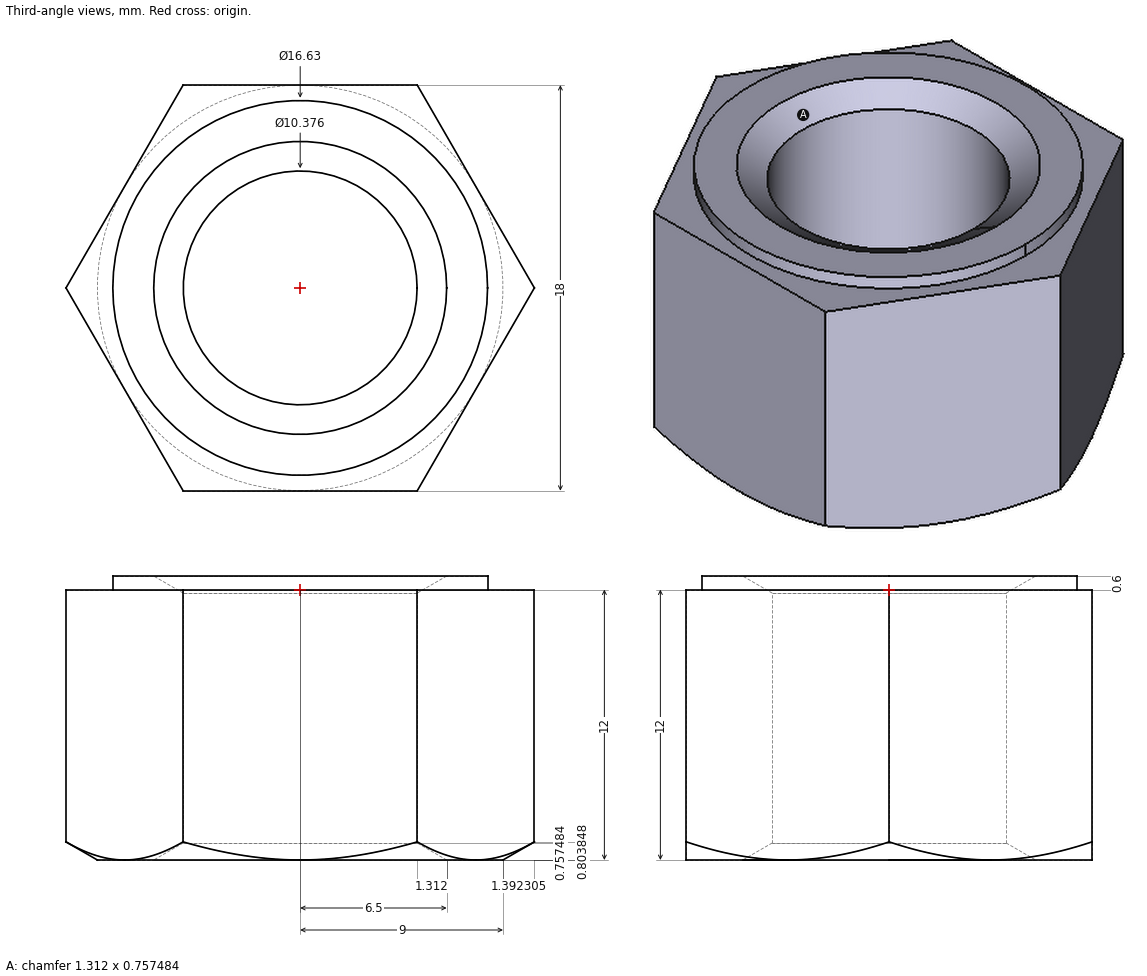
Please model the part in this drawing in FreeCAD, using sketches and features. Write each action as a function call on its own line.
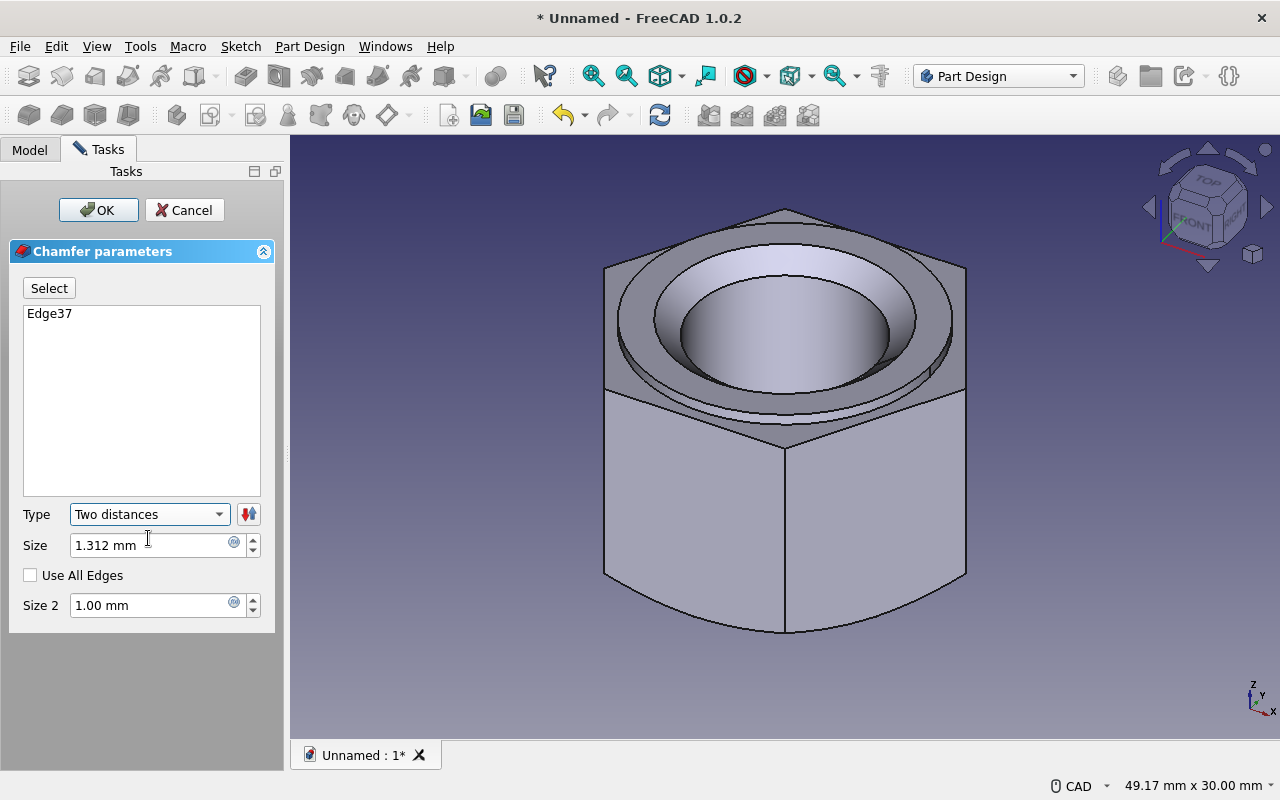
triple_click(158, 606)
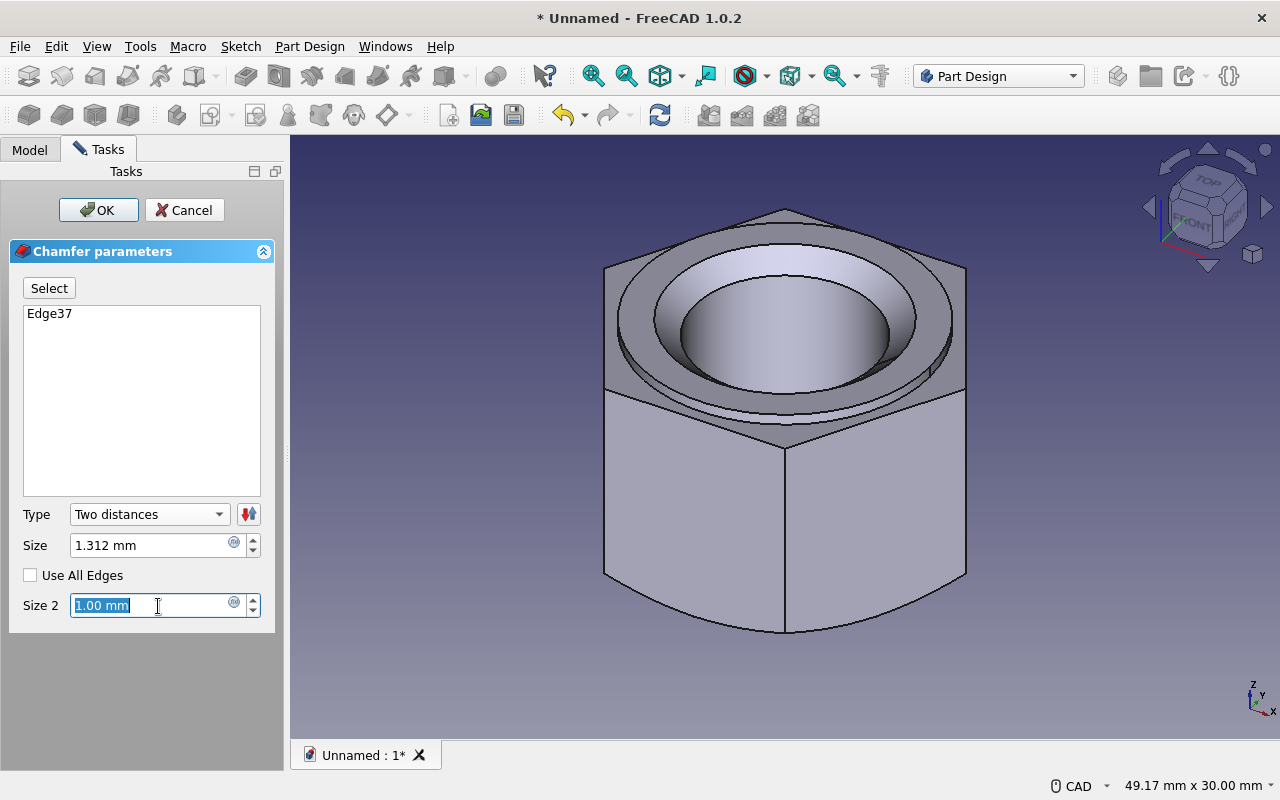
text(0.757484)
key(Tab)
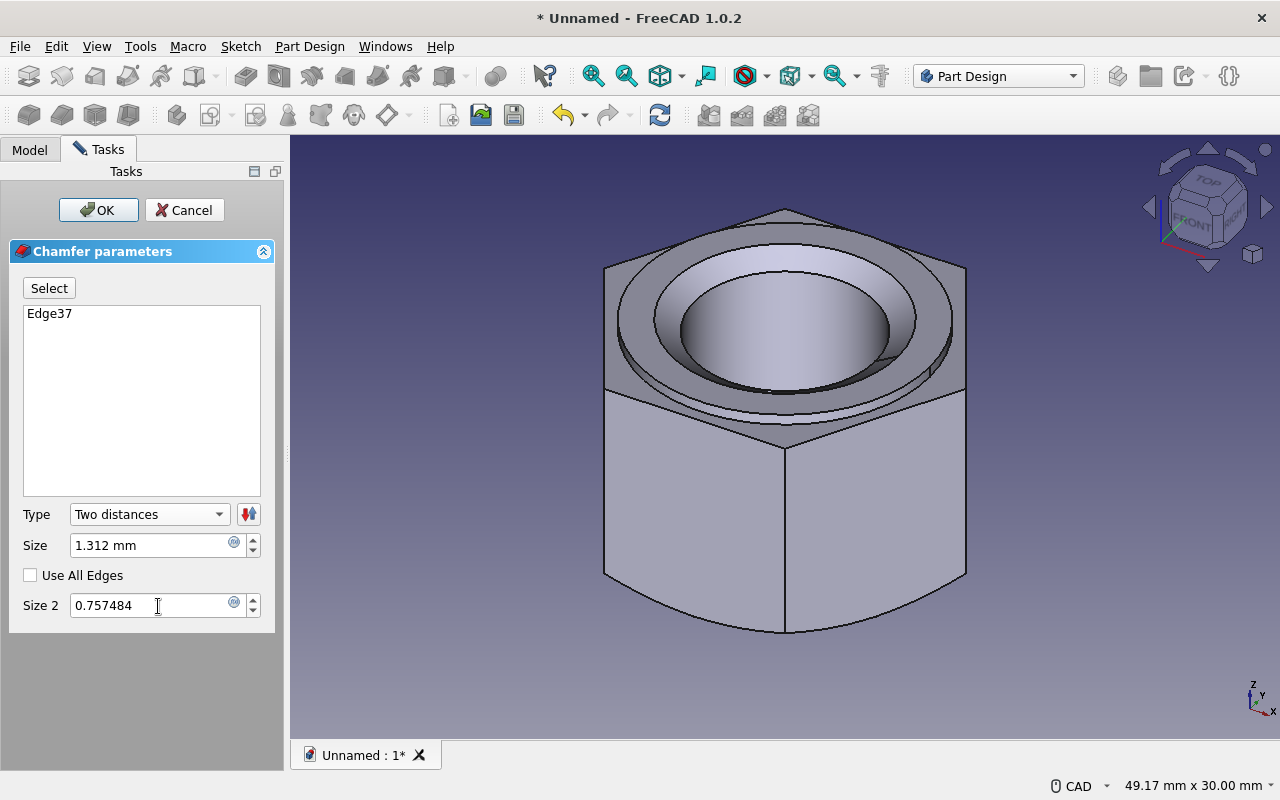
click(99, 210)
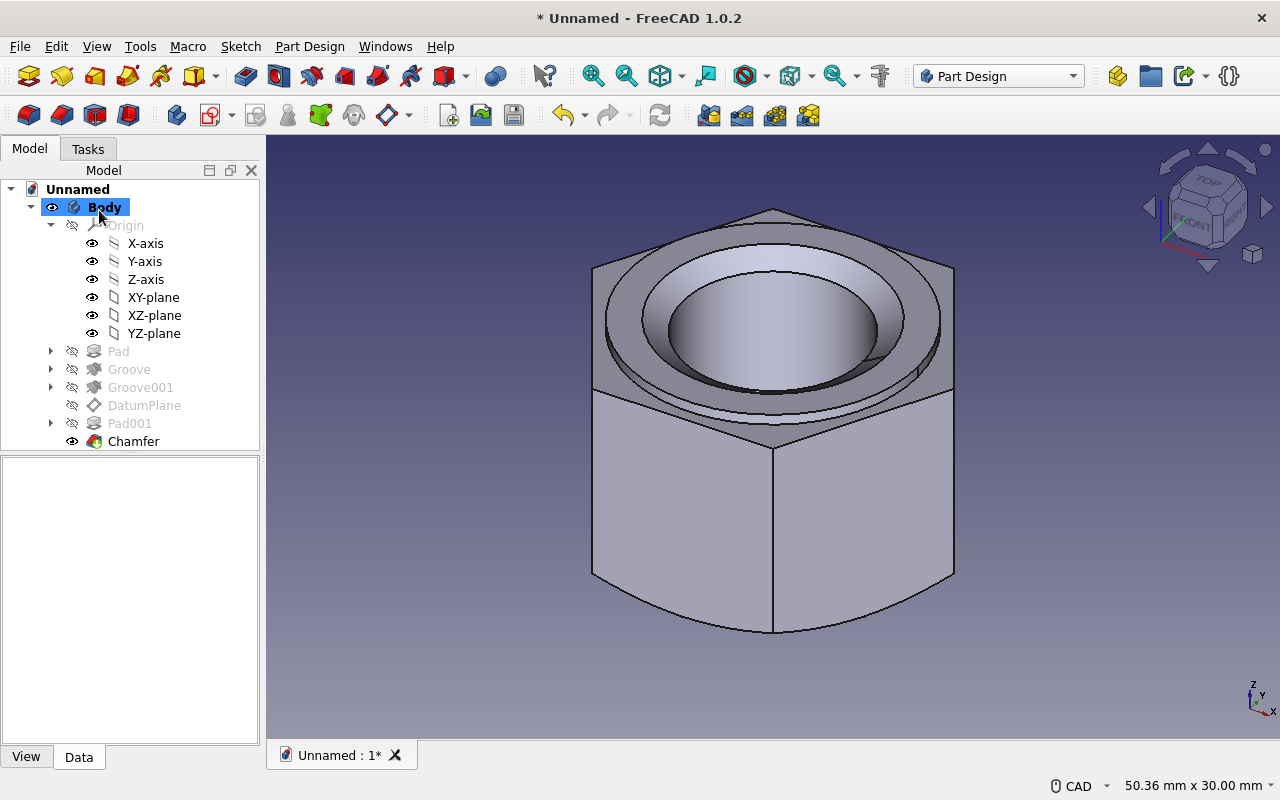
key(0)